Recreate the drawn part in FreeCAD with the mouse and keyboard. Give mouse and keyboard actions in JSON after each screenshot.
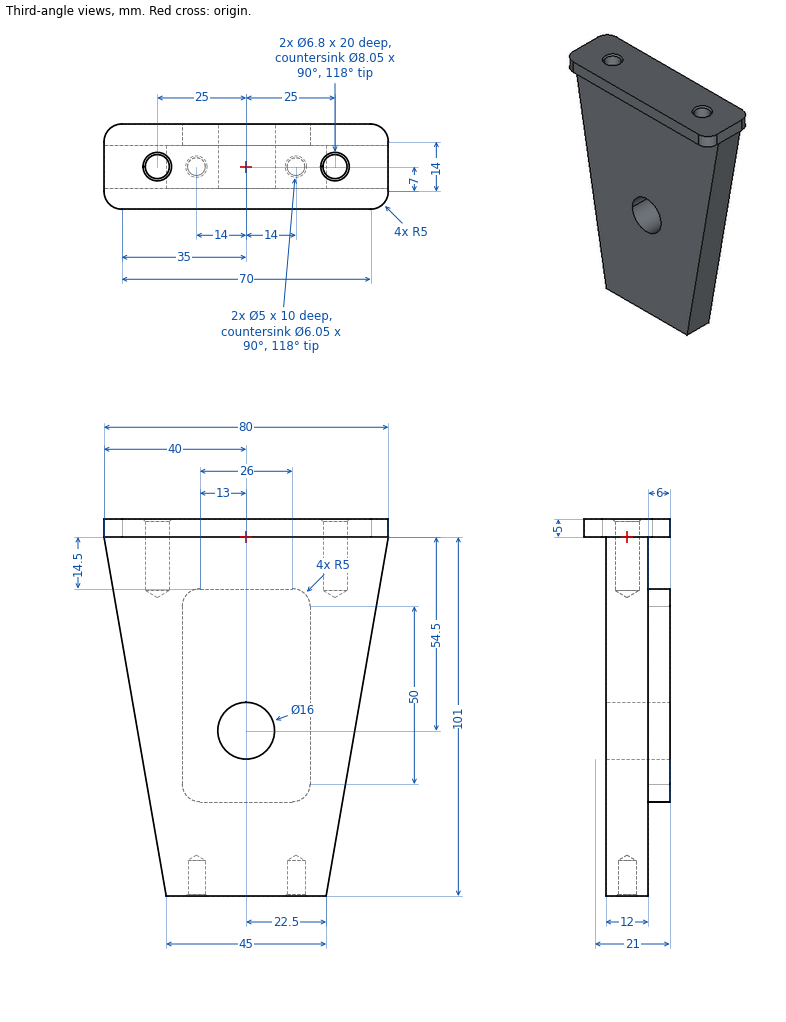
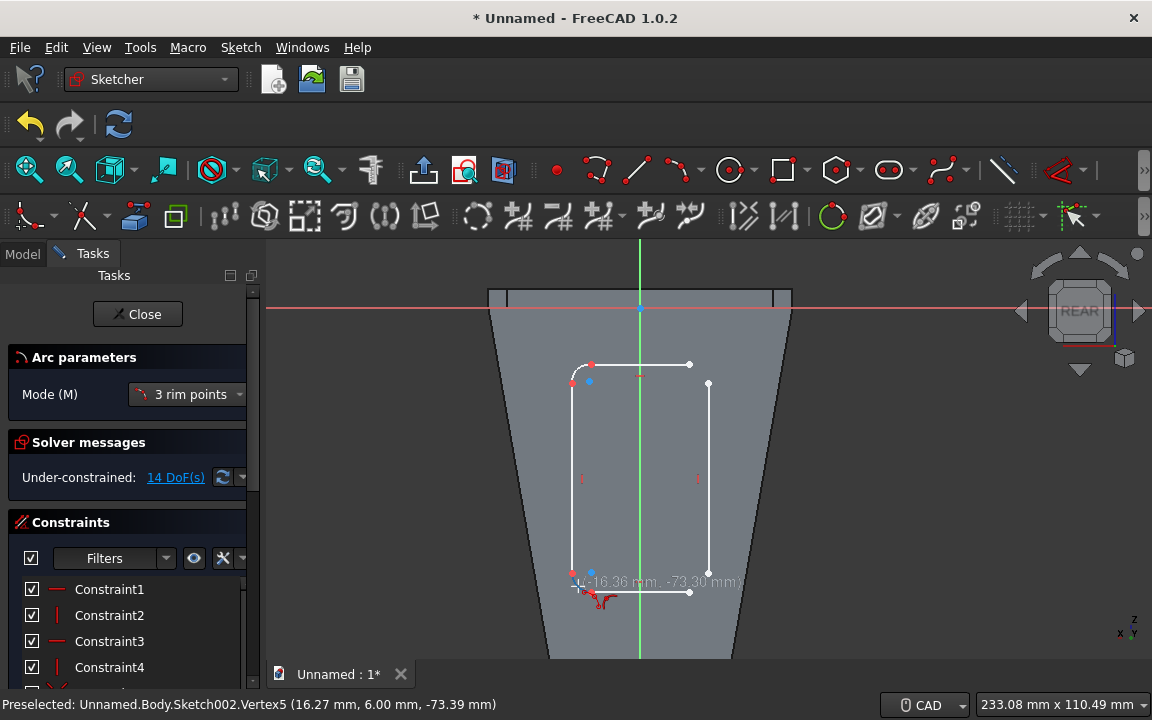
{"action": "left_click", "coordinate": [689, 592]}
{"action": "left_click", "coordinate": [709, 574]}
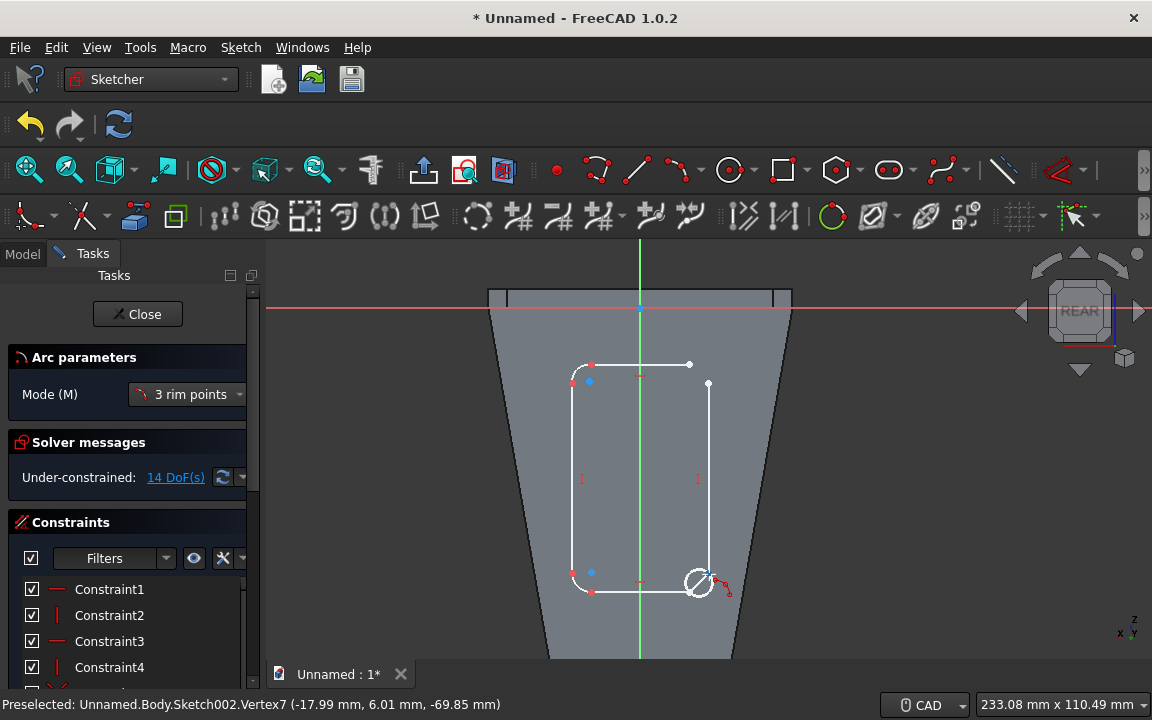
{"action": "scroll", "coordinate": [703, 586], "scroll_direction": "up", "scroll_amount": 6}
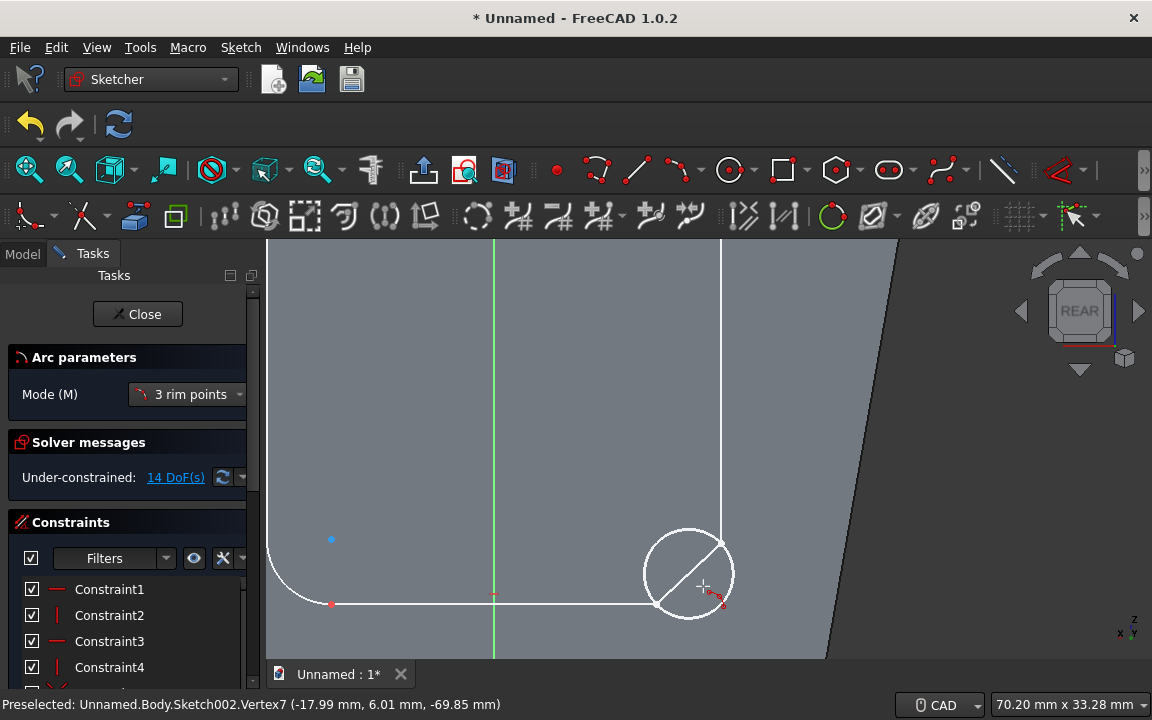
{"action": "left_click", "coordinate": [703, 584]}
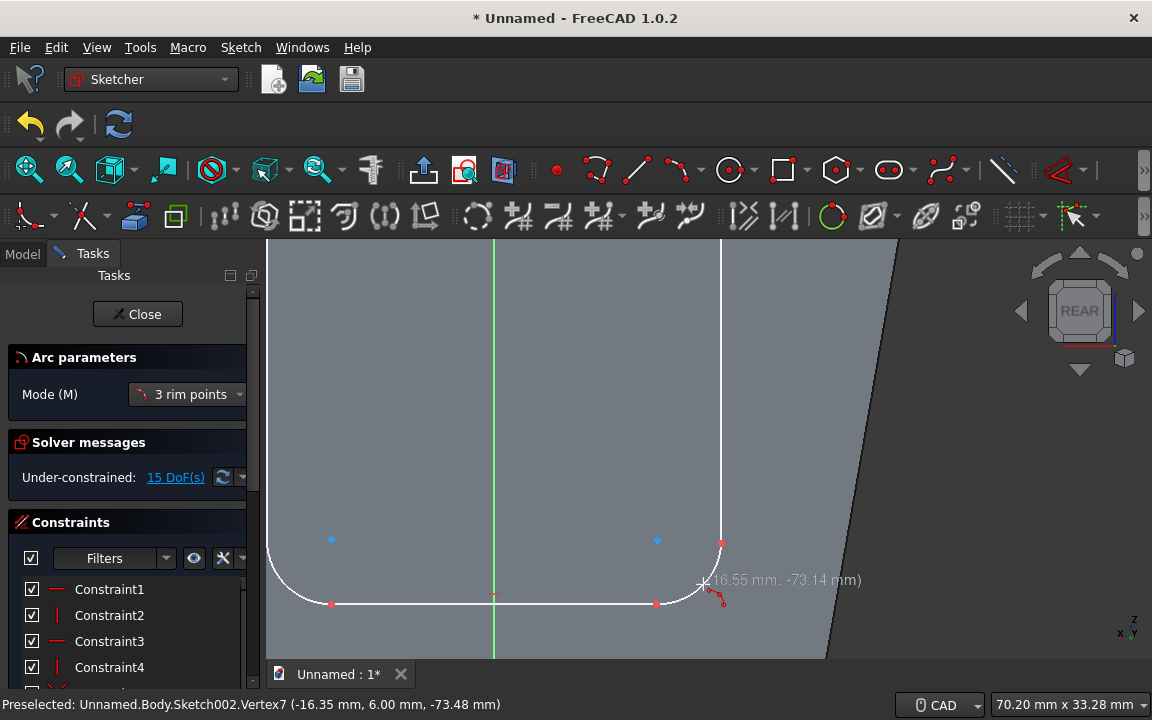
{"action": "scroll", "coordinate": [704, 586], "scroll_direction": "down", "scroll_amount": 6}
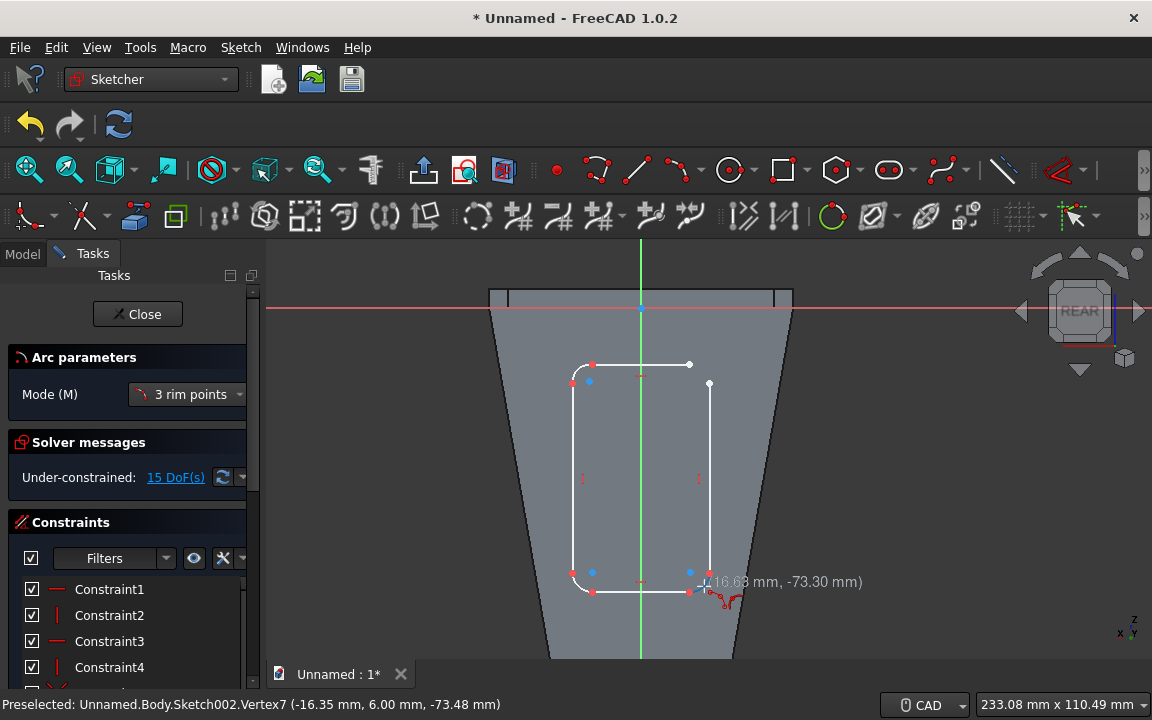
{"action": "left_click", "coordinate": [710, 383]}
{"action": "left_click", "coordinate": [690, 365]}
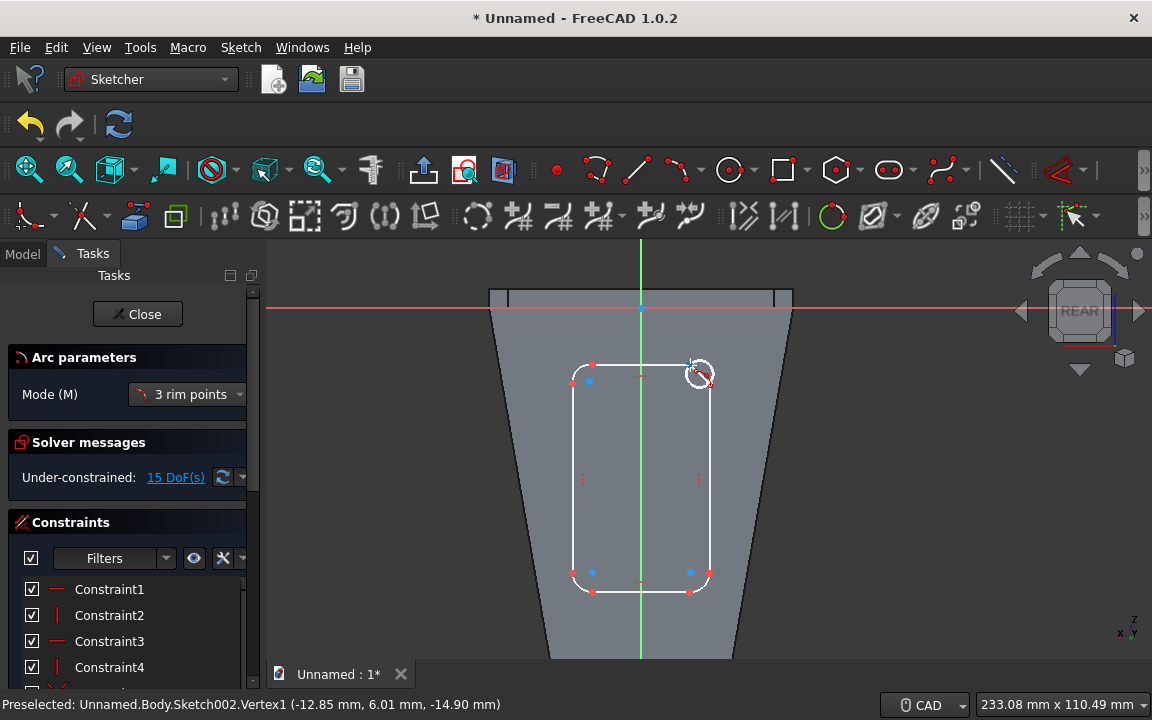
{"action": "scroll", "coordinate": [704, 369], "scroll_direction": "up", "scroll_amount": 6}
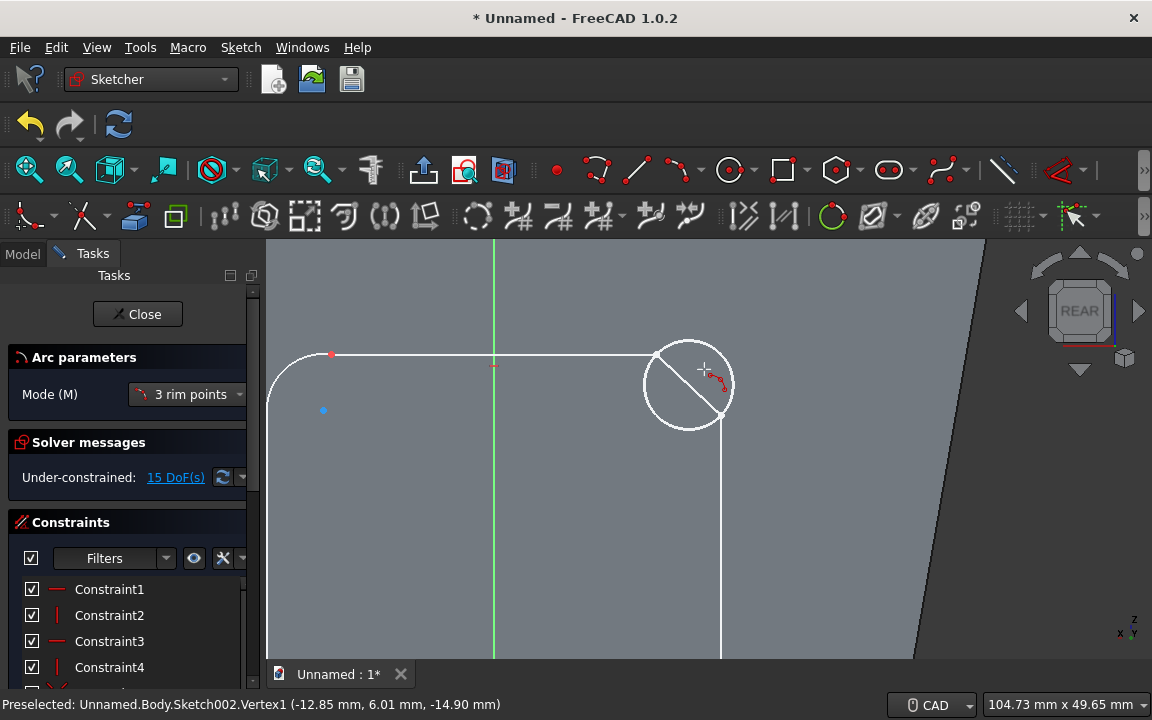
{"action": "left_click", "coordinate": [703, 368]}
{"action": "key", "text": "Escape"}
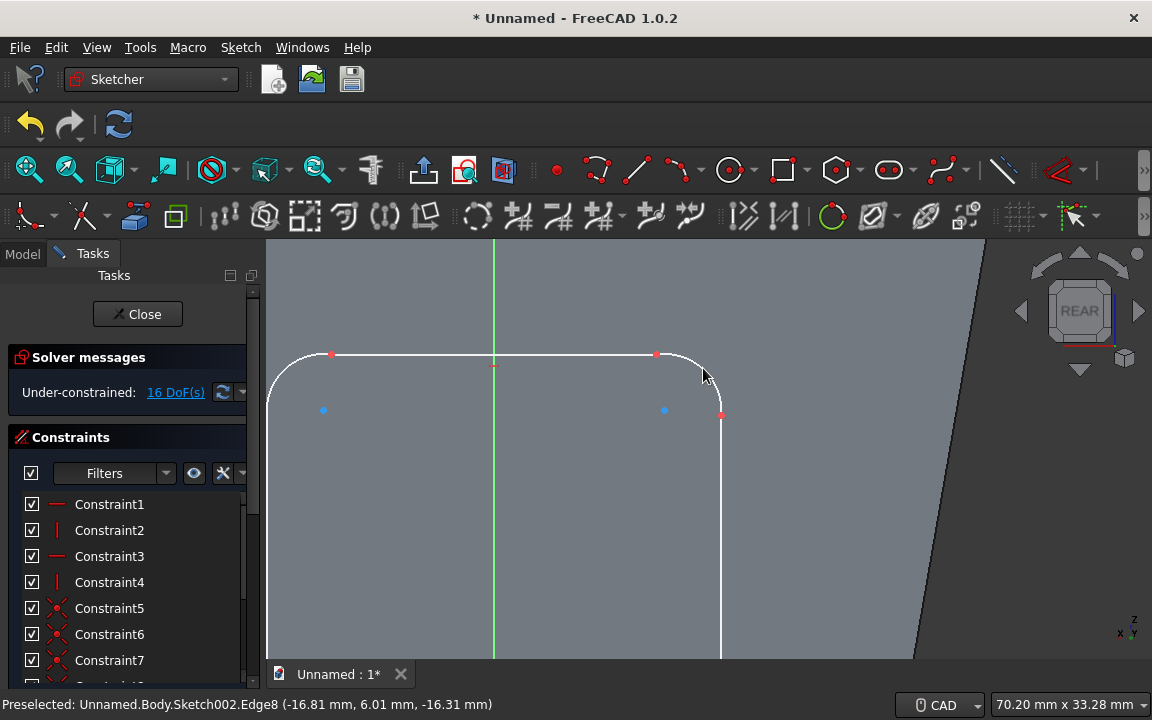
{"action": "scroll", "coordinate": [704, 368], "scroll_direction": "down", "scroll_amount": 6}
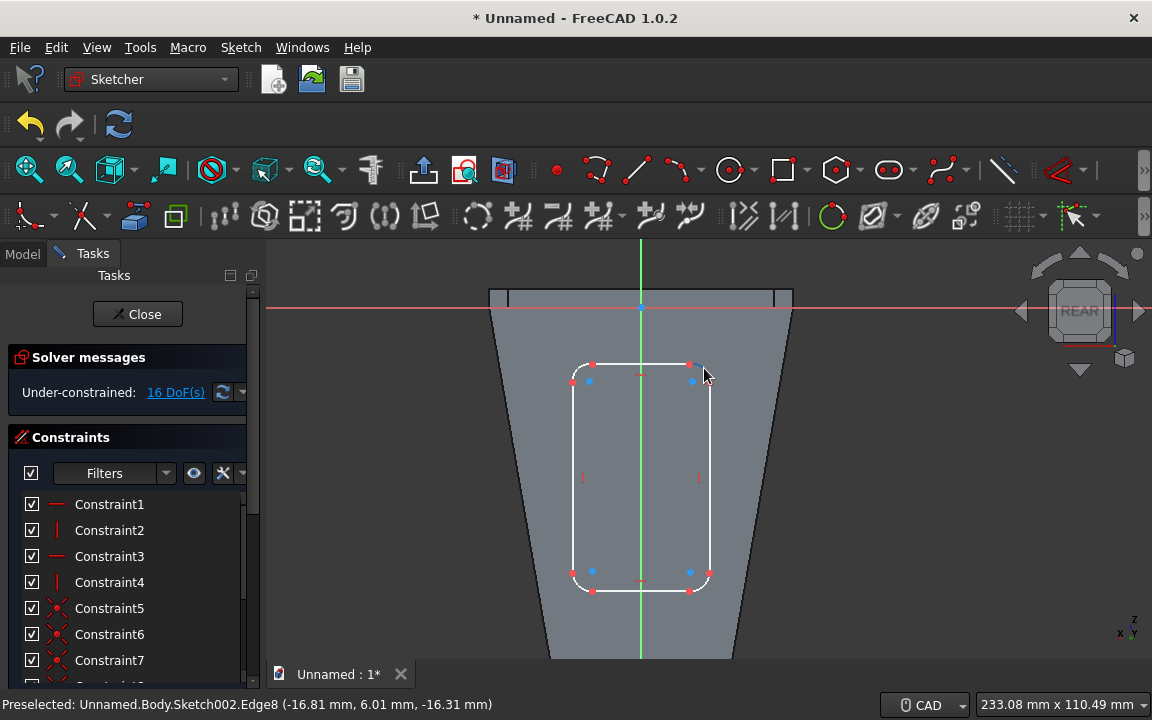
{"action": "left_click", "coordinate": [661, 364]}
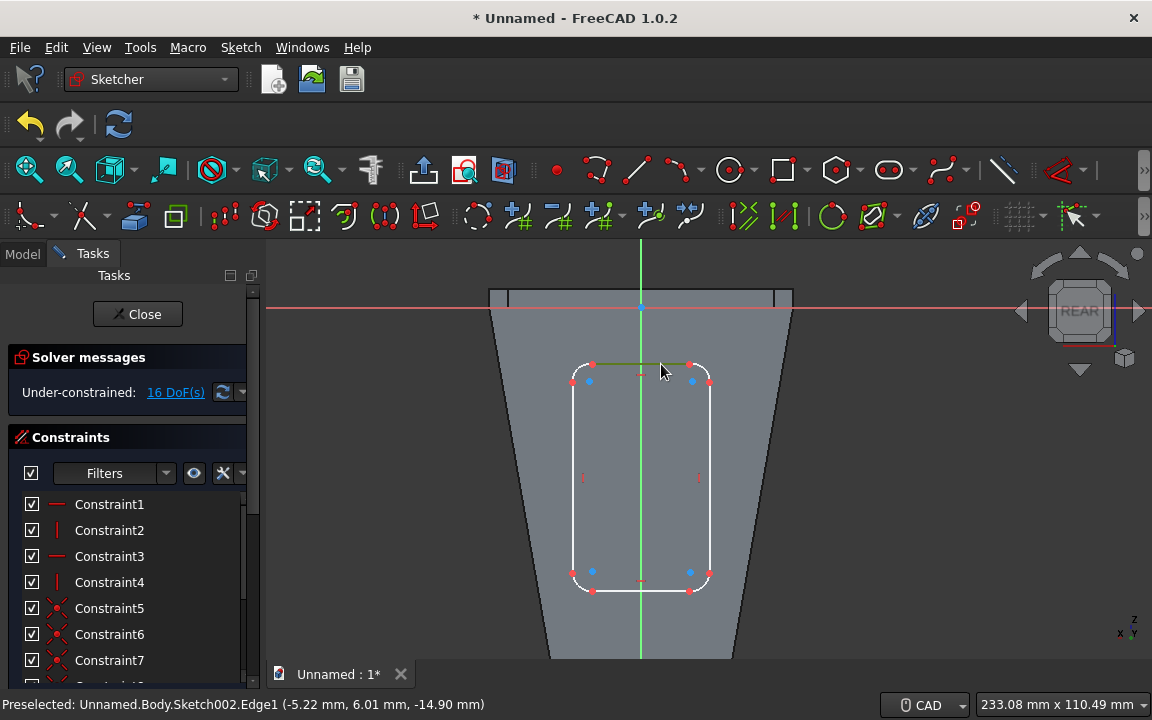
{"action": "scroll", "coordinate": [583, 365], "scroll_direction": "up", "scroll_amount": 3}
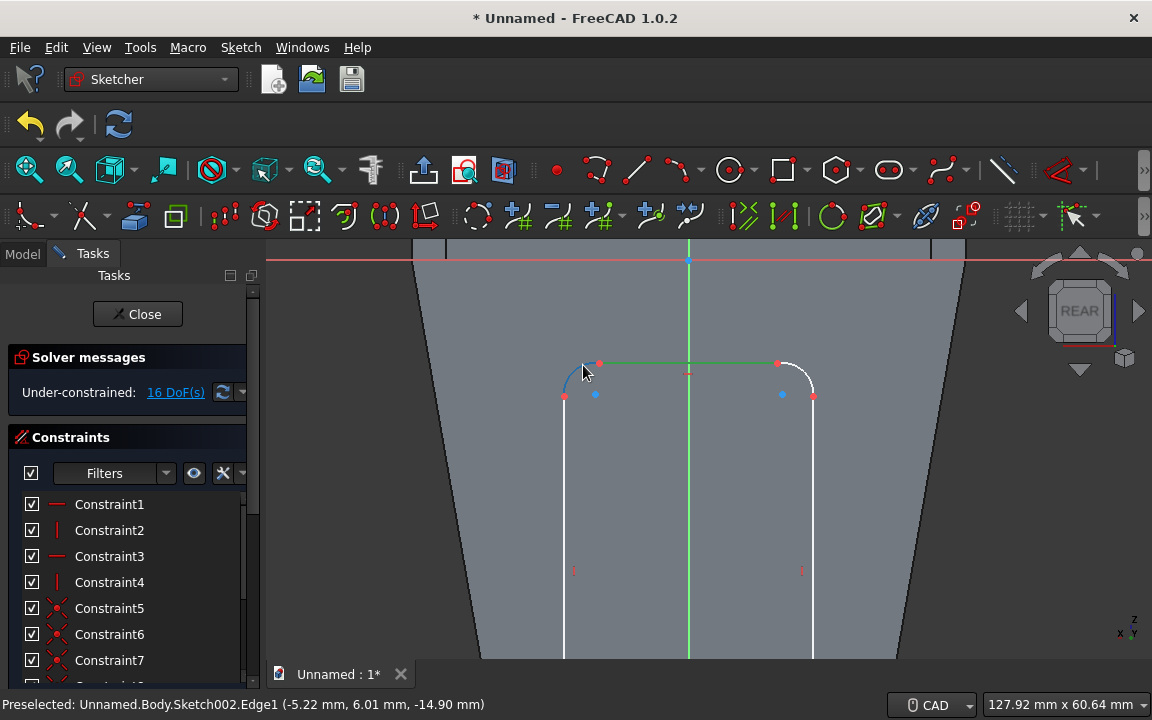
{"action": "left_click", "coordinate": [583, 365]}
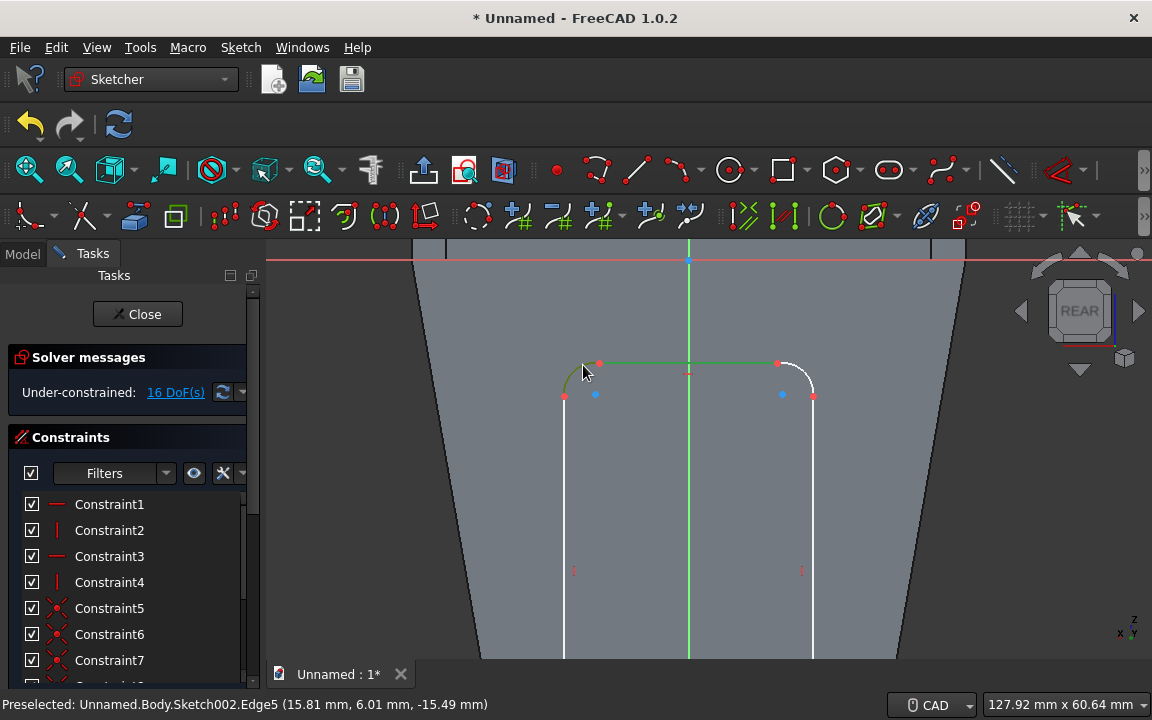
{"action": "key", "text": "t"}